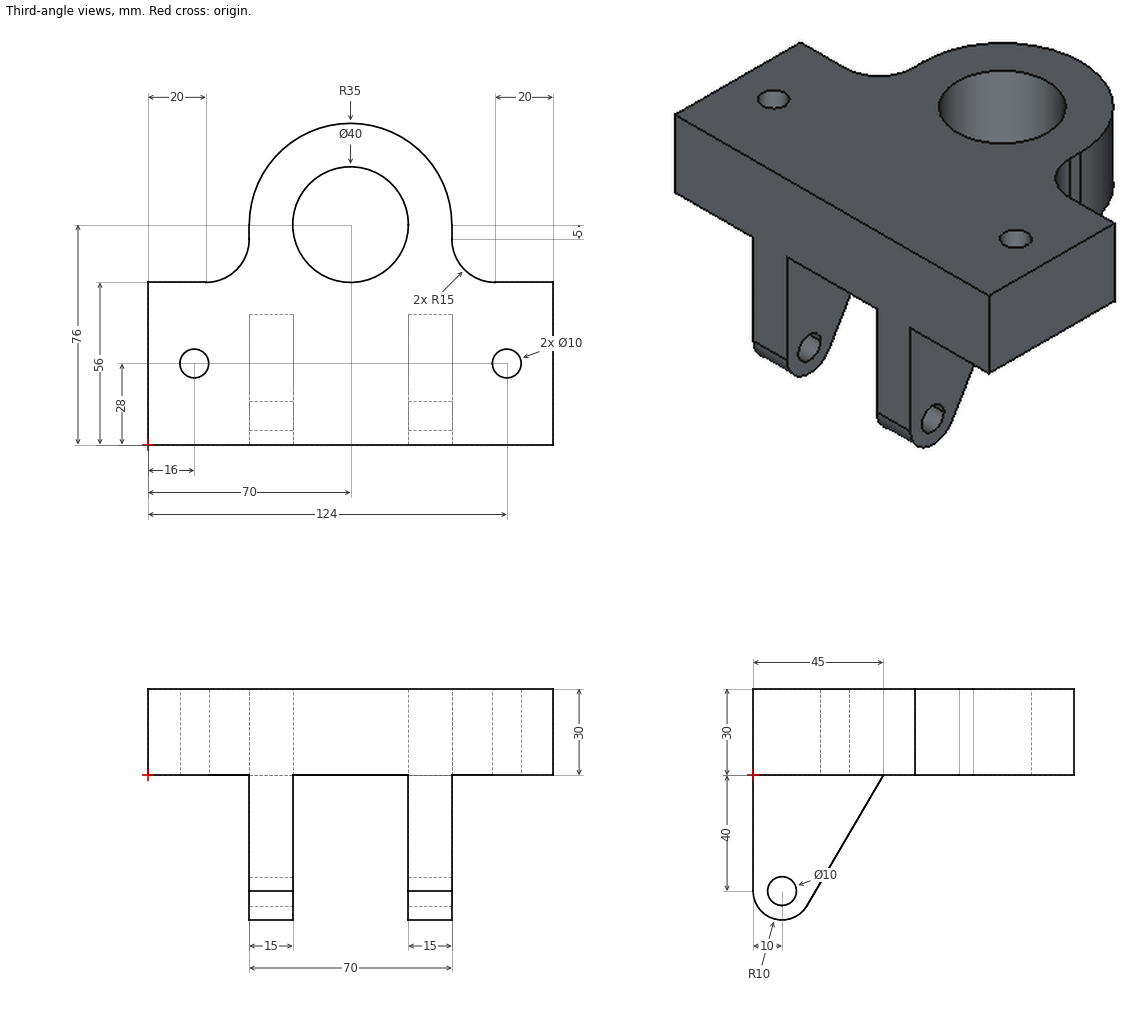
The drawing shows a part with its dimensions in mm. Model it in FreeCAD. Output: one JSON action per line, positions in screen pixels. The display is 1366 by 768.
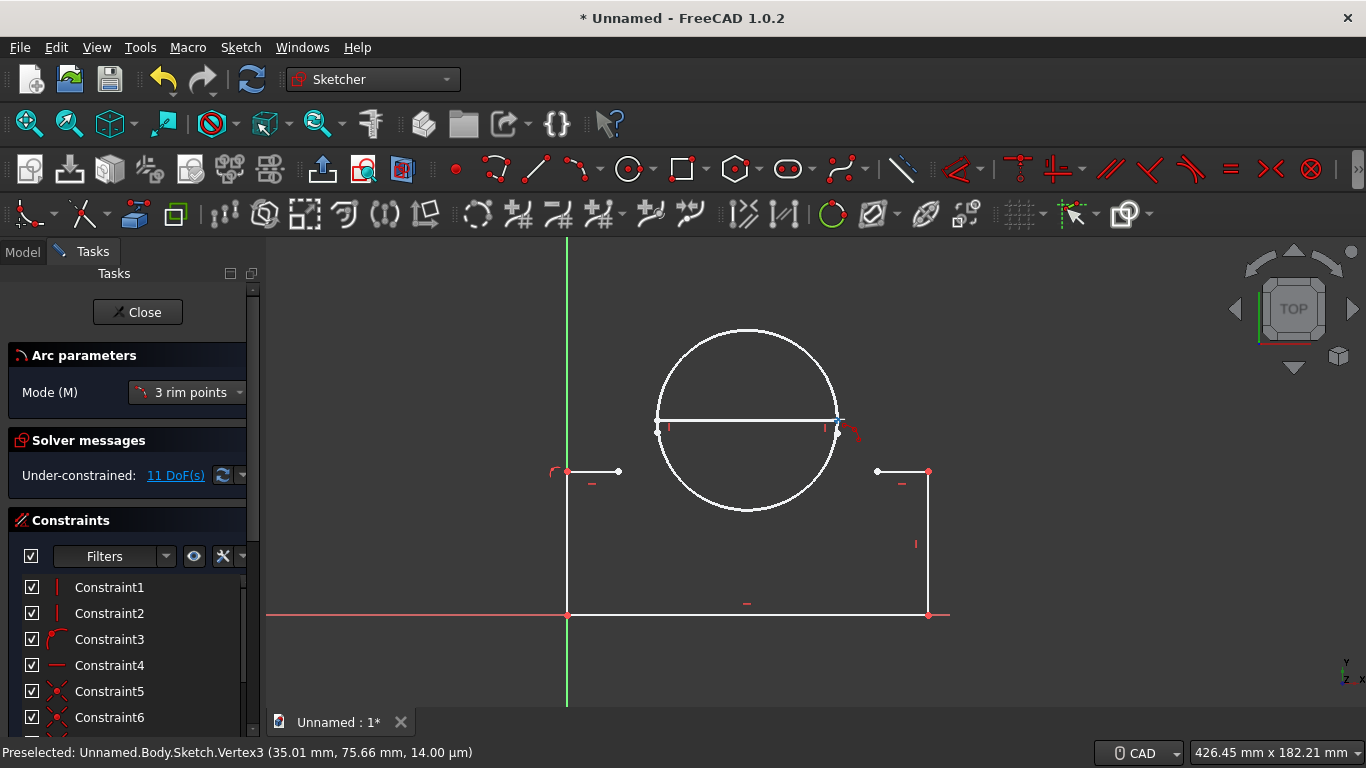
{"action": "left_click", "coordinate": [748, 329]}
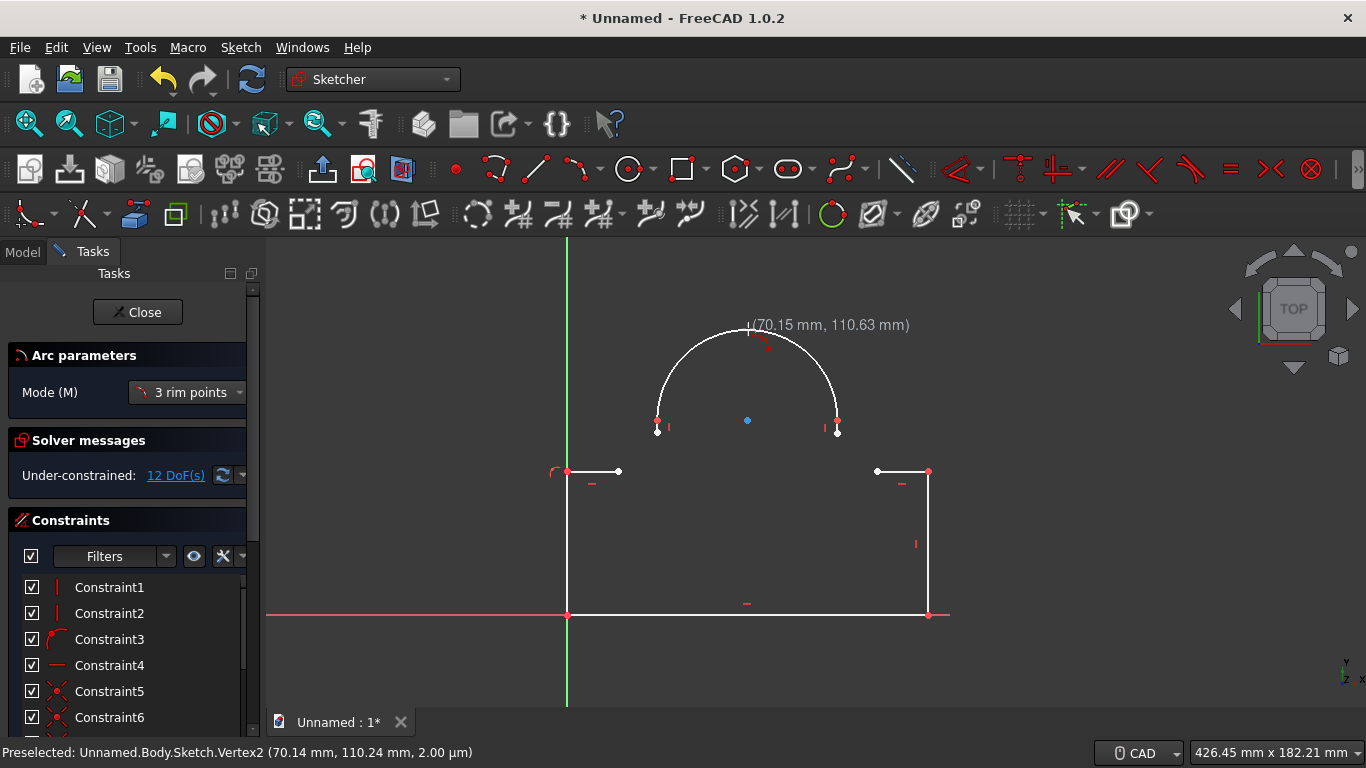
{"action": "scroll", "coordinate": [657, 432], "scroll_direction": "up", "scroll_amount": 5}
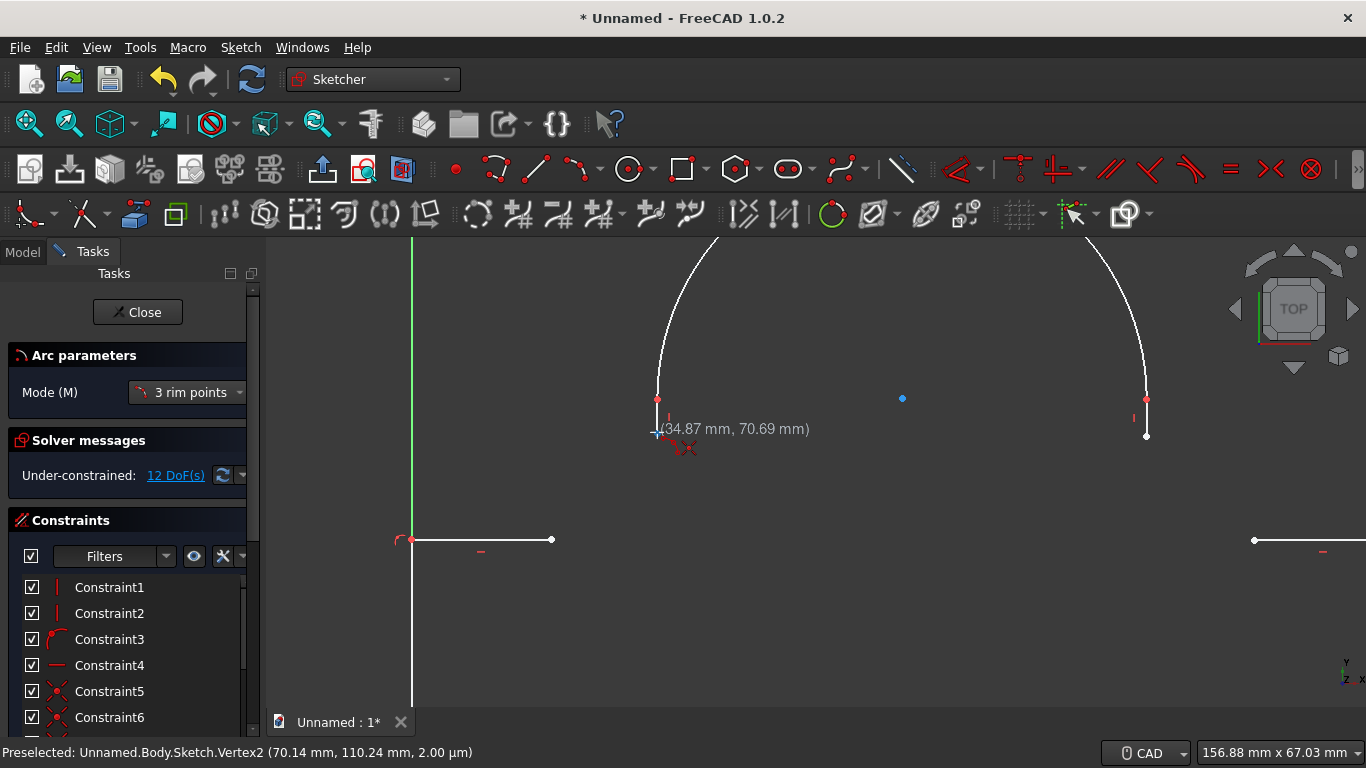
{"action": "left_click", "coordinate": [657, 434]}
{"action": "left_click", "coordinate": [552, 540]}
{"action": "left_click", "coordinate": [626, 506]}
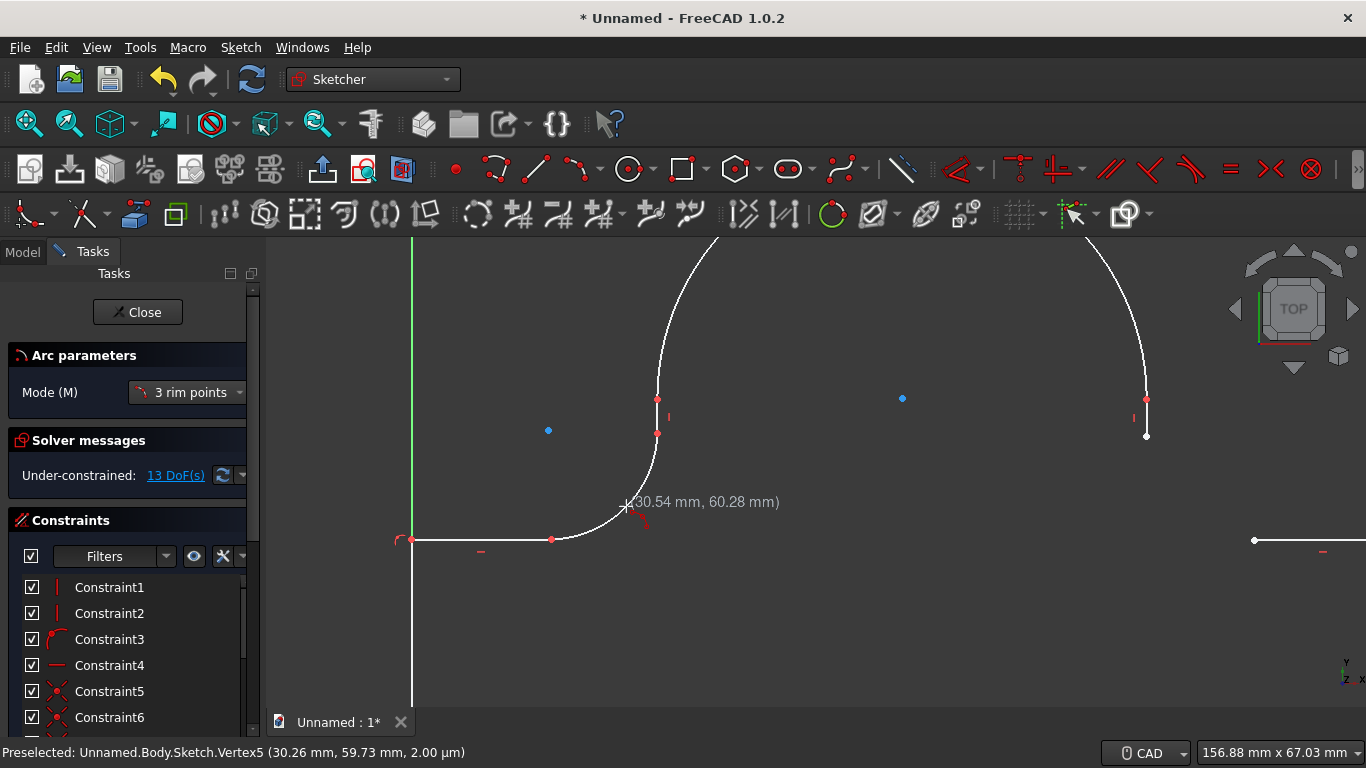
{"action": "scroll", "coordinate": [657, 432], "scroll_direction": "down", "scroll_amount": 5}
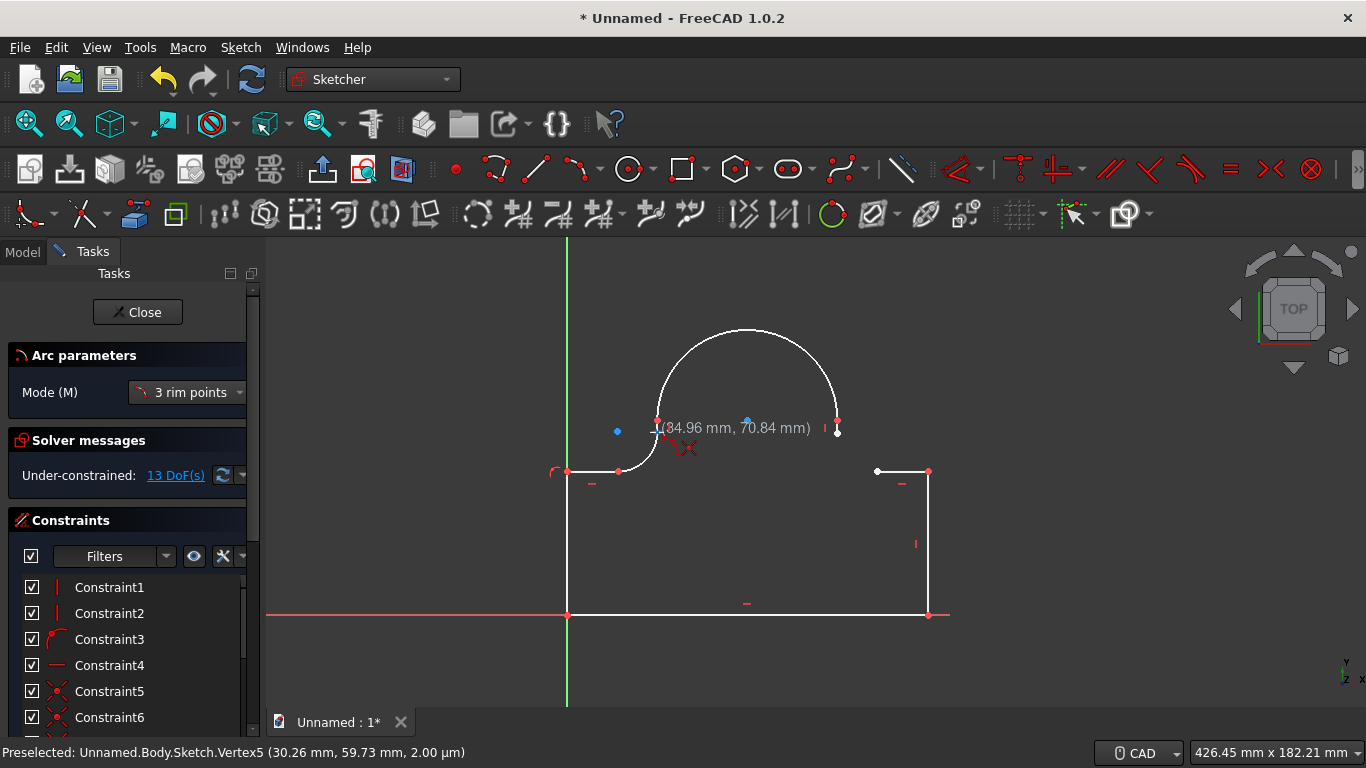
{"action": "left_click", "coordinate": [877, 472]}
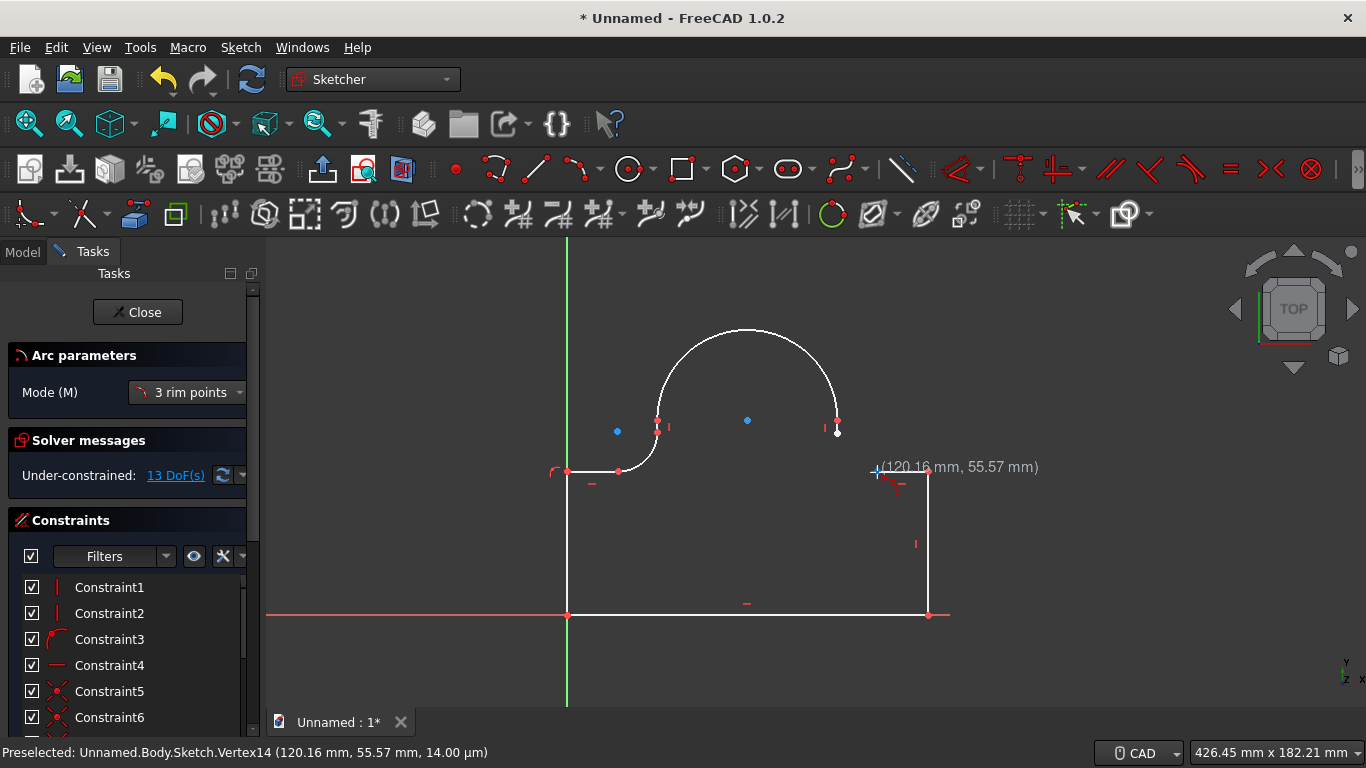
{"action": "scroll", "coordinate": [838, 432], "scroll_direction": "up", "scroll_amount": 5}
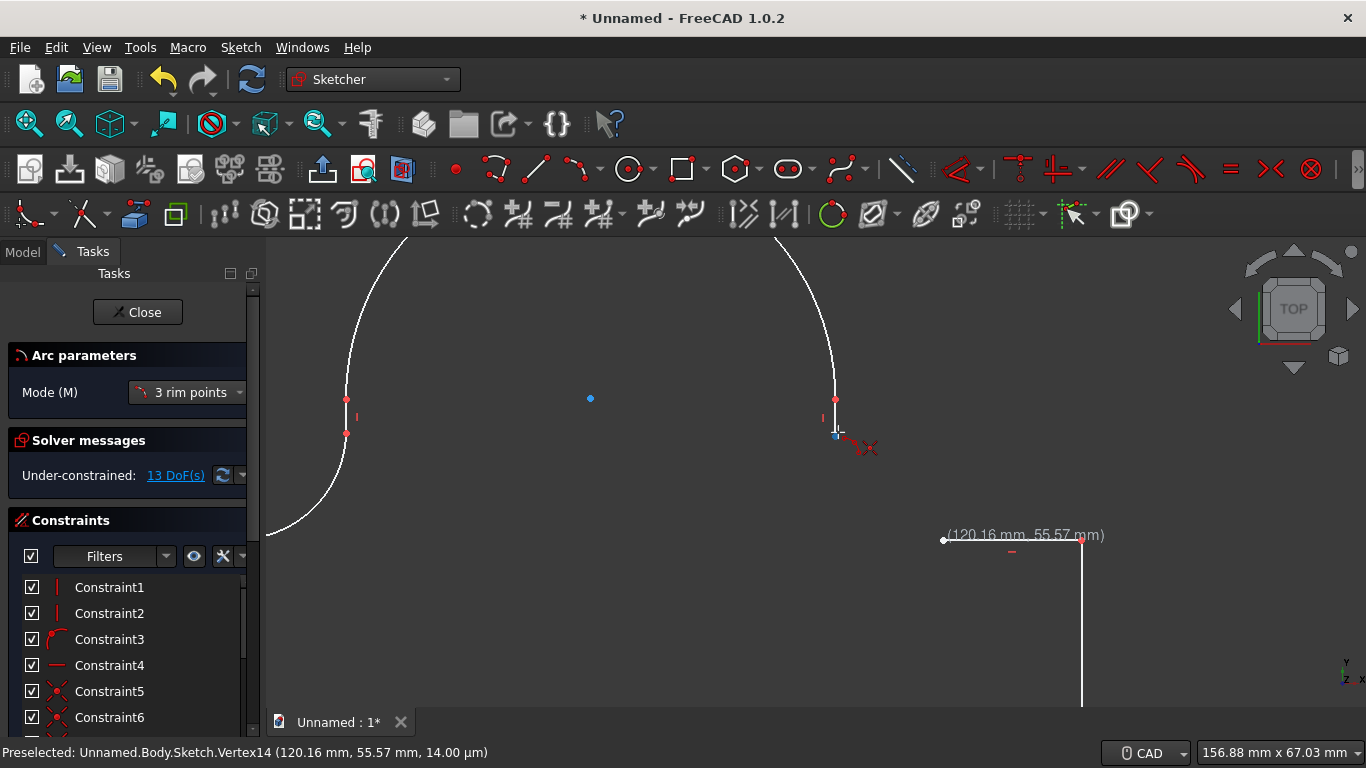
{"action": "left_click", "coordinate": [835, 437]}
{"action": "left_click", "coordinate": [868, 506]}
{"action": "key", "text": "Escape"}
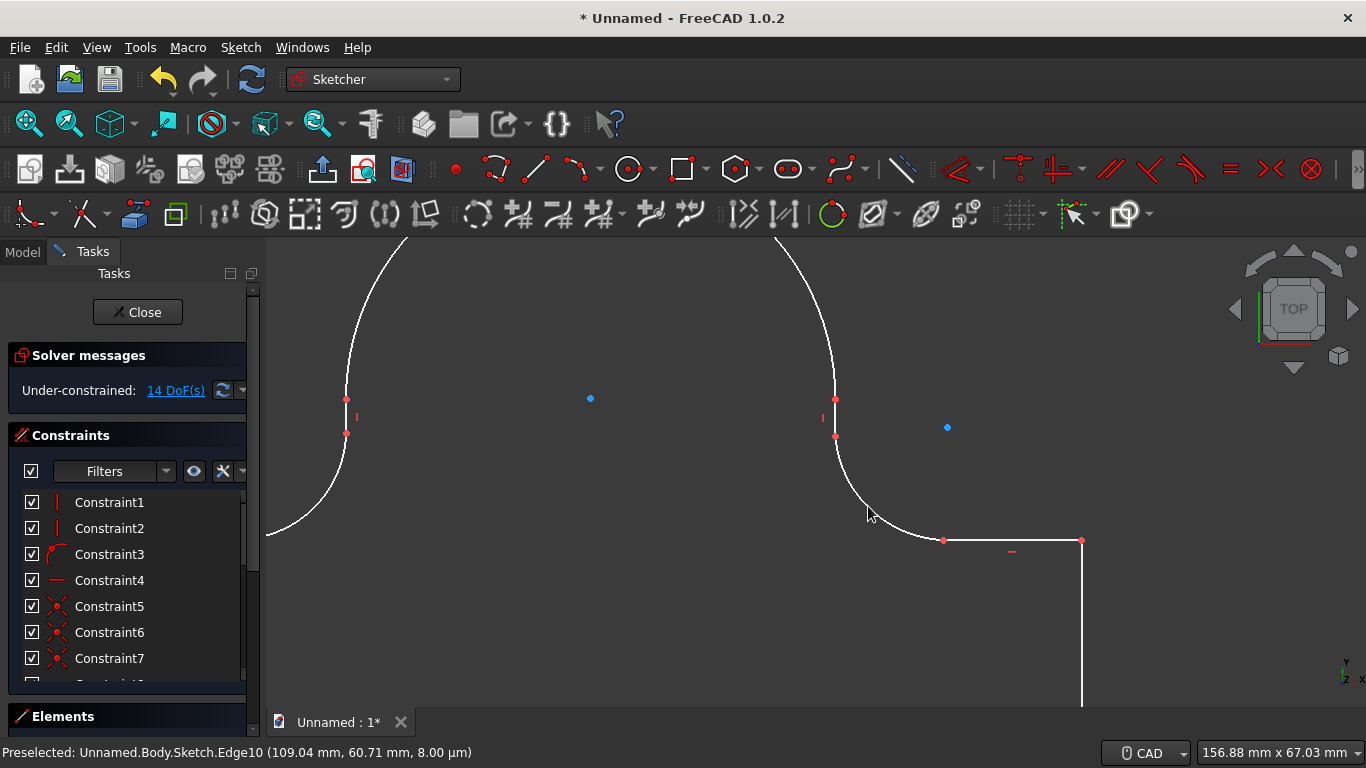
{"action": "scroll", "coordinate": [835, 425], "scroll_direction": "up", "scroll_amount": 2}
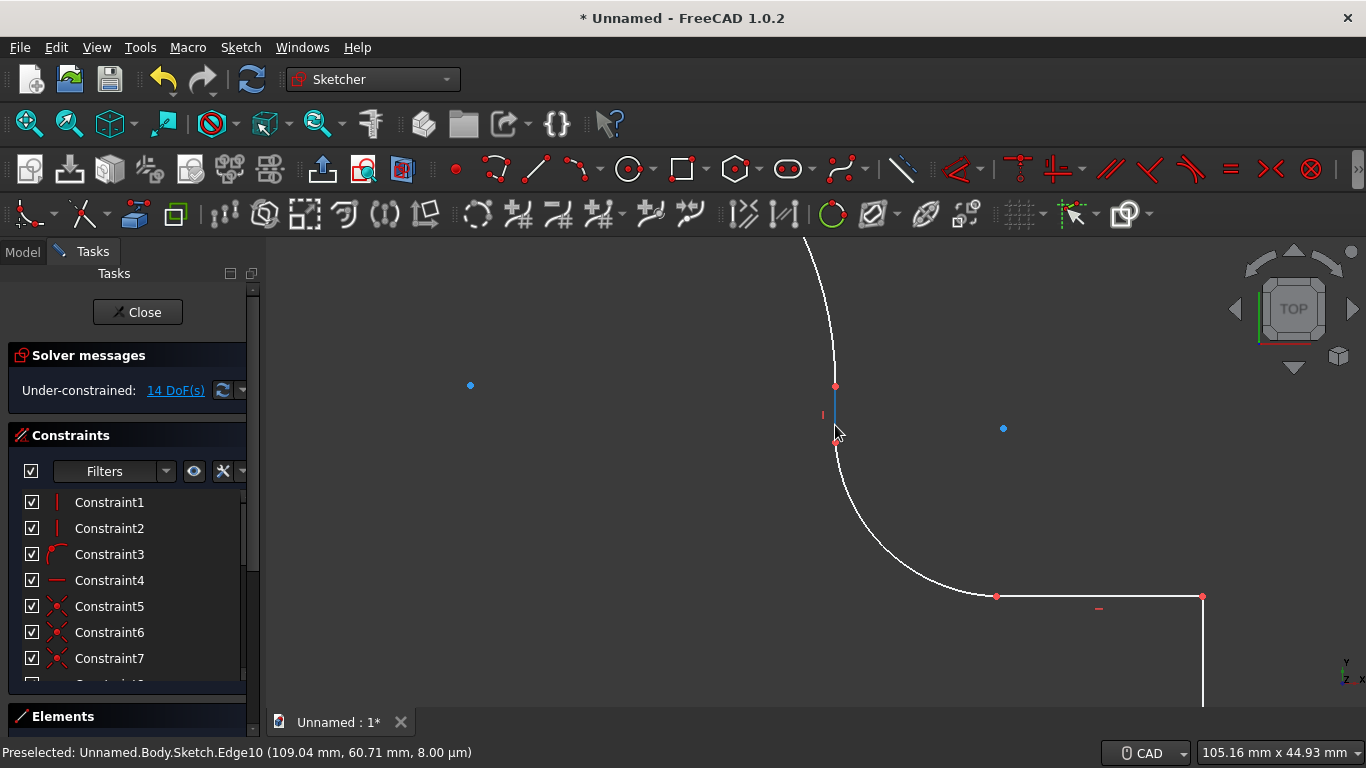
{"action": "left_click", "coordinate": [835, 425]}